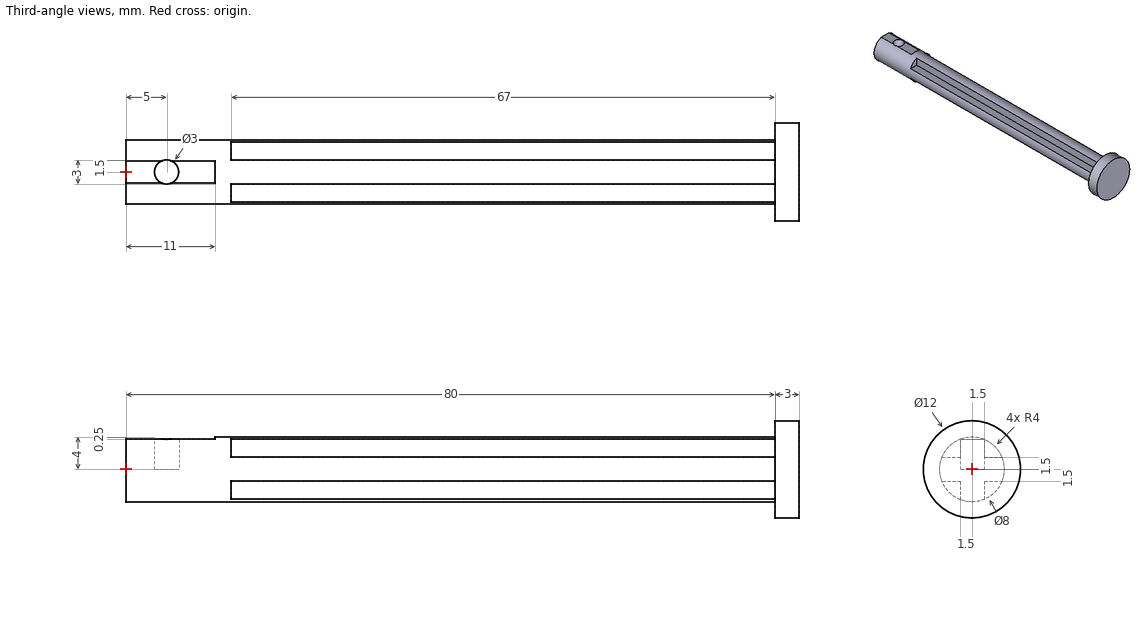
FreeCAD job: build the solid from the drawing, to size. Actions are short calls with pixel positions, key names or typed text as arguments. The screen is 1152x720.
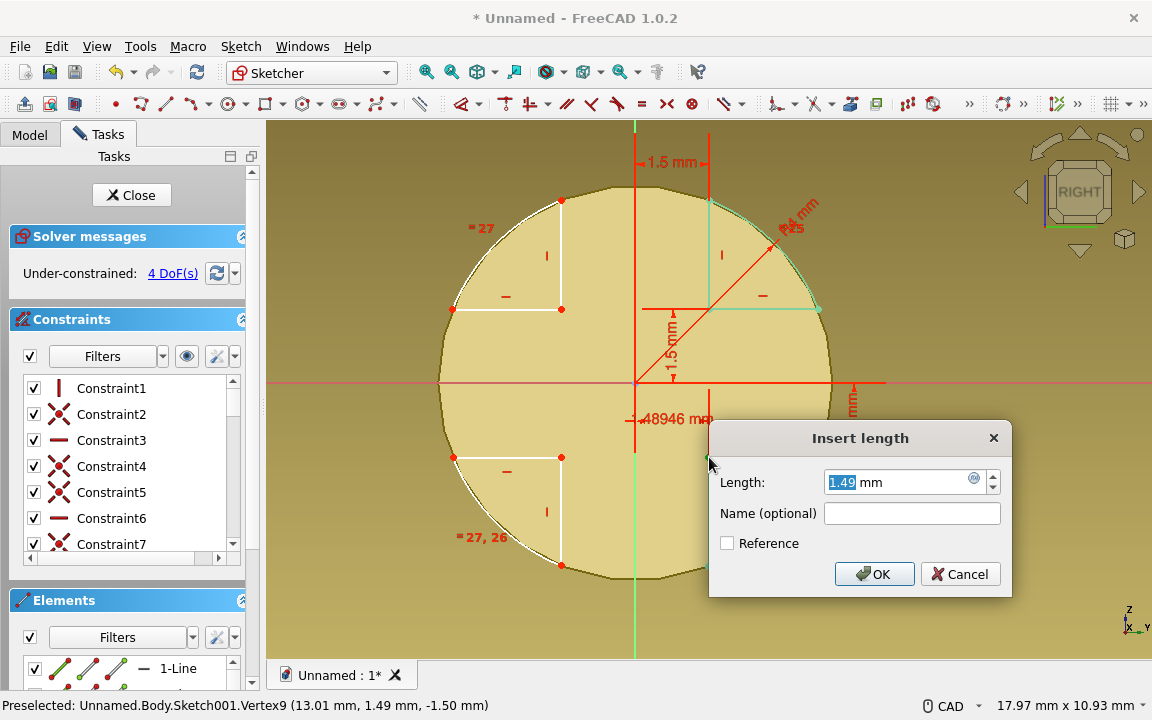
text(1.5)
key(Return)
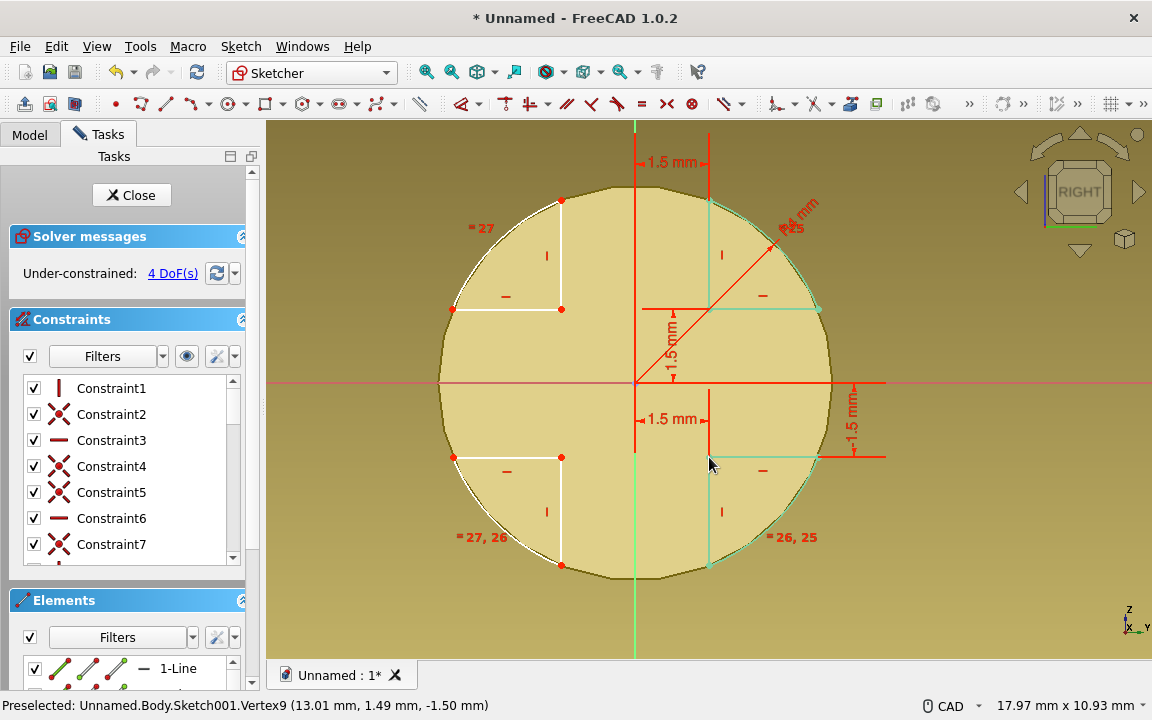
click(561, 566)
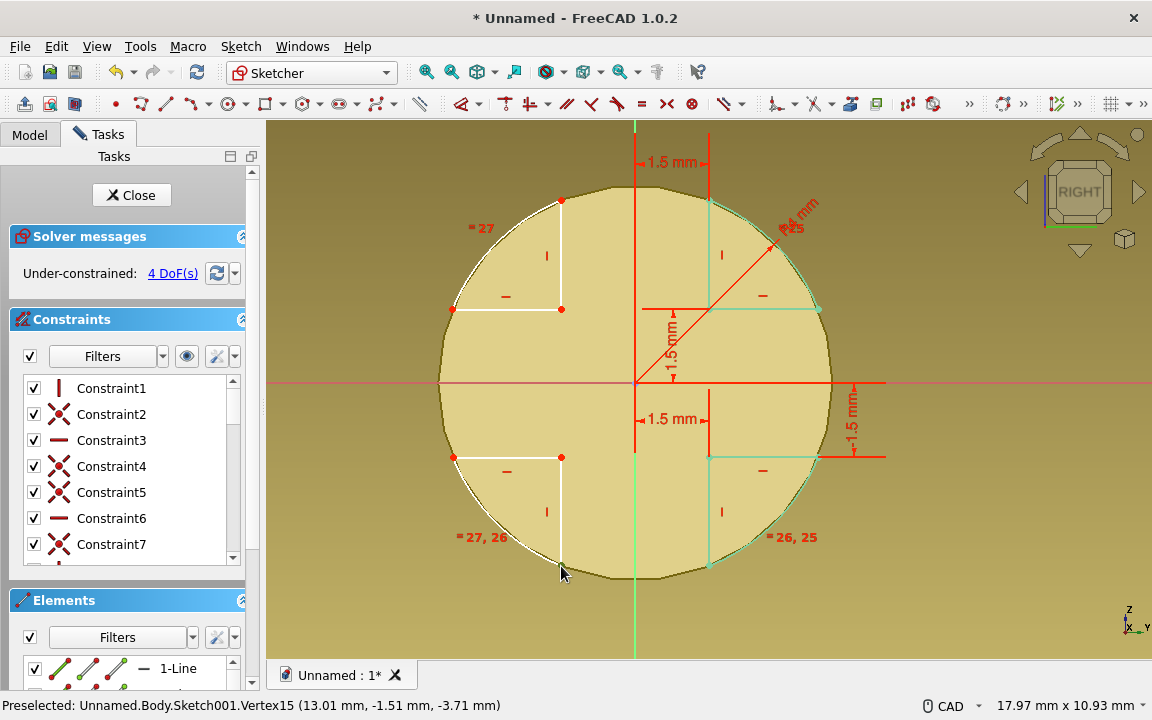
key(l)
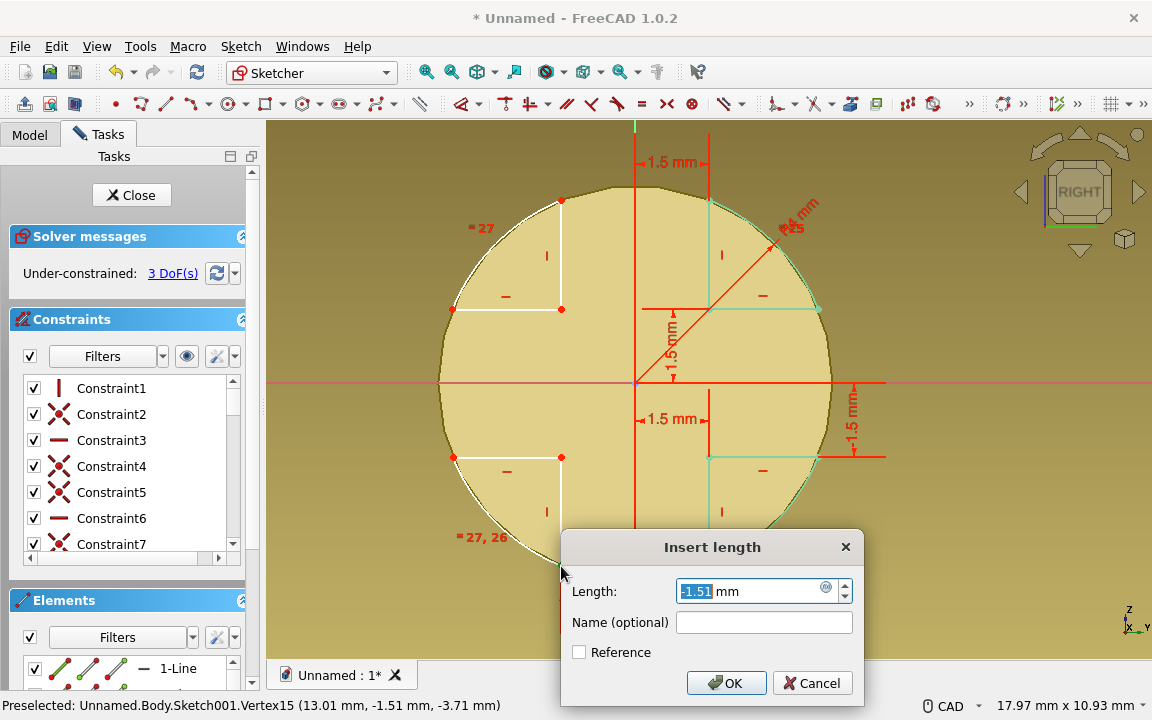
text(-1.5)
key(Return)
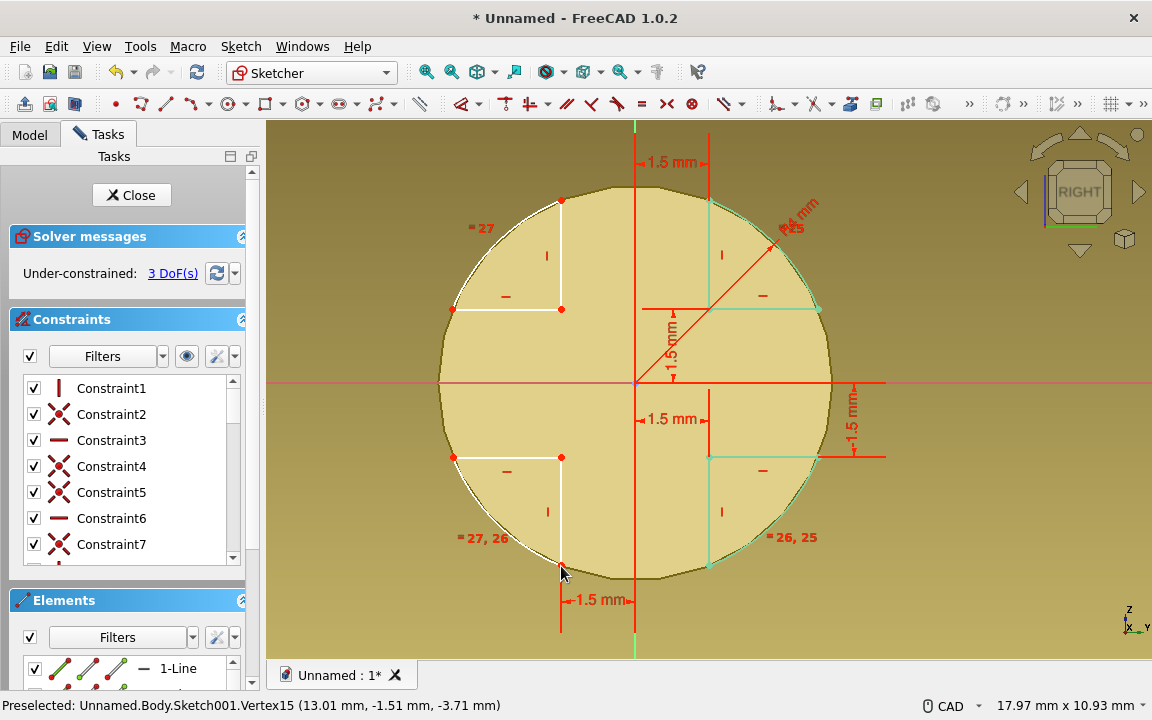
click(561, 458)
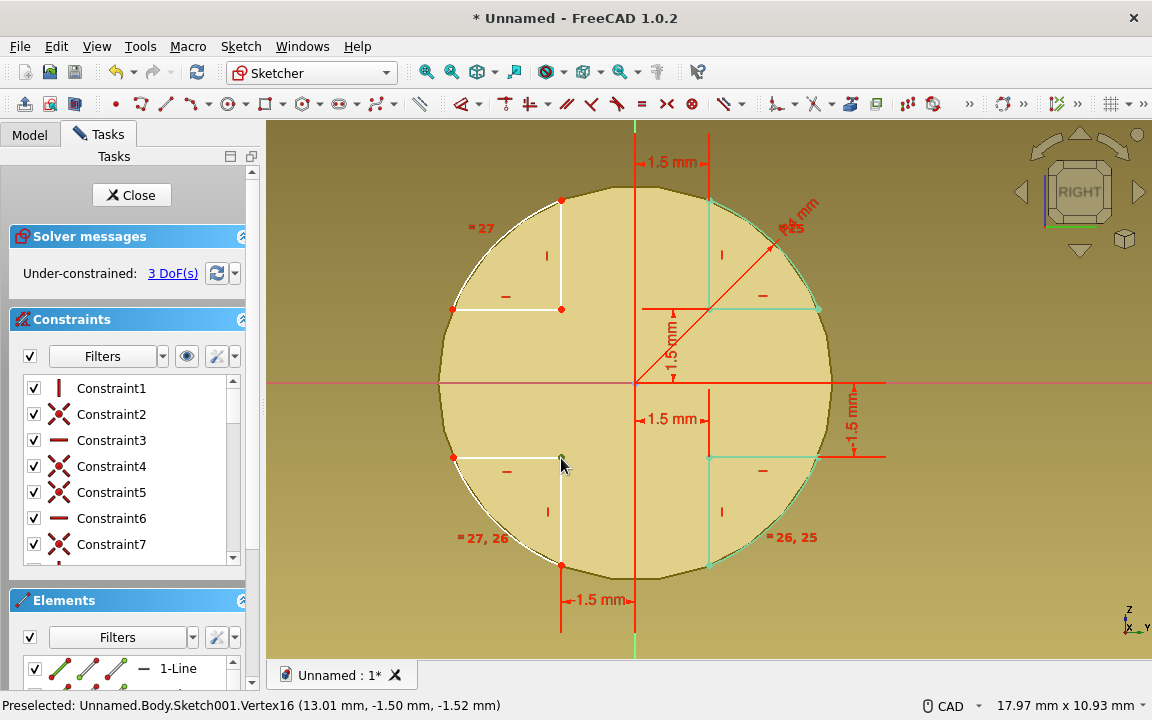
key(i)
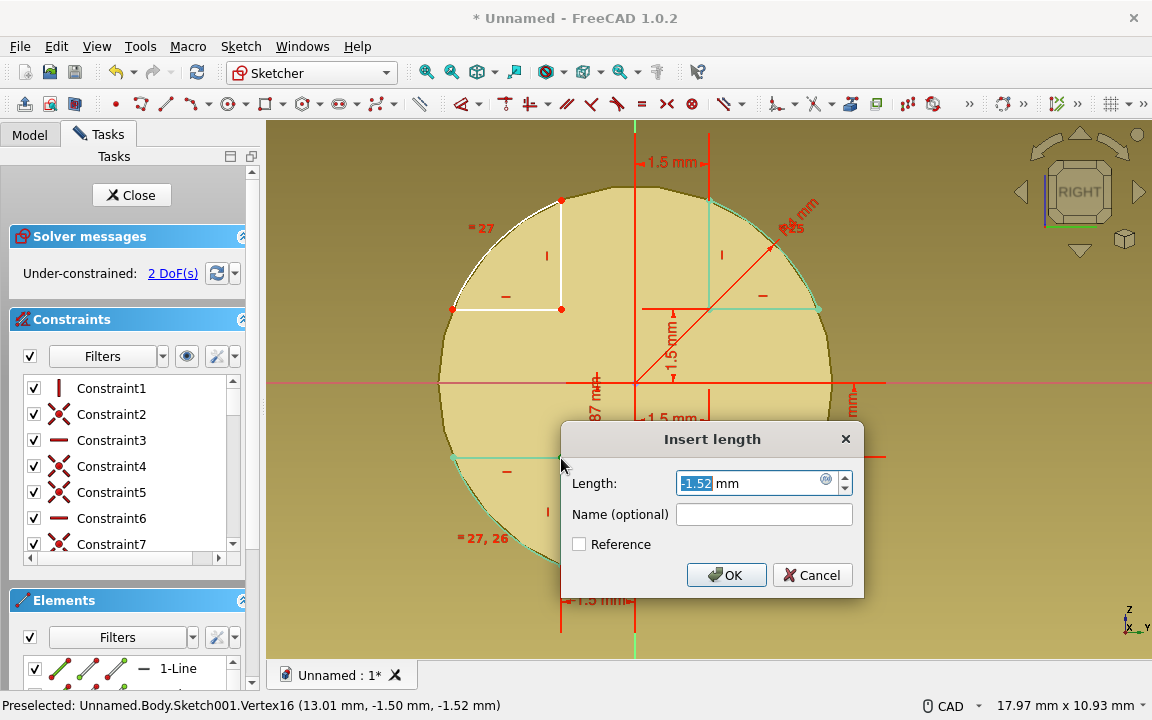
text(-1.5)
key(Return)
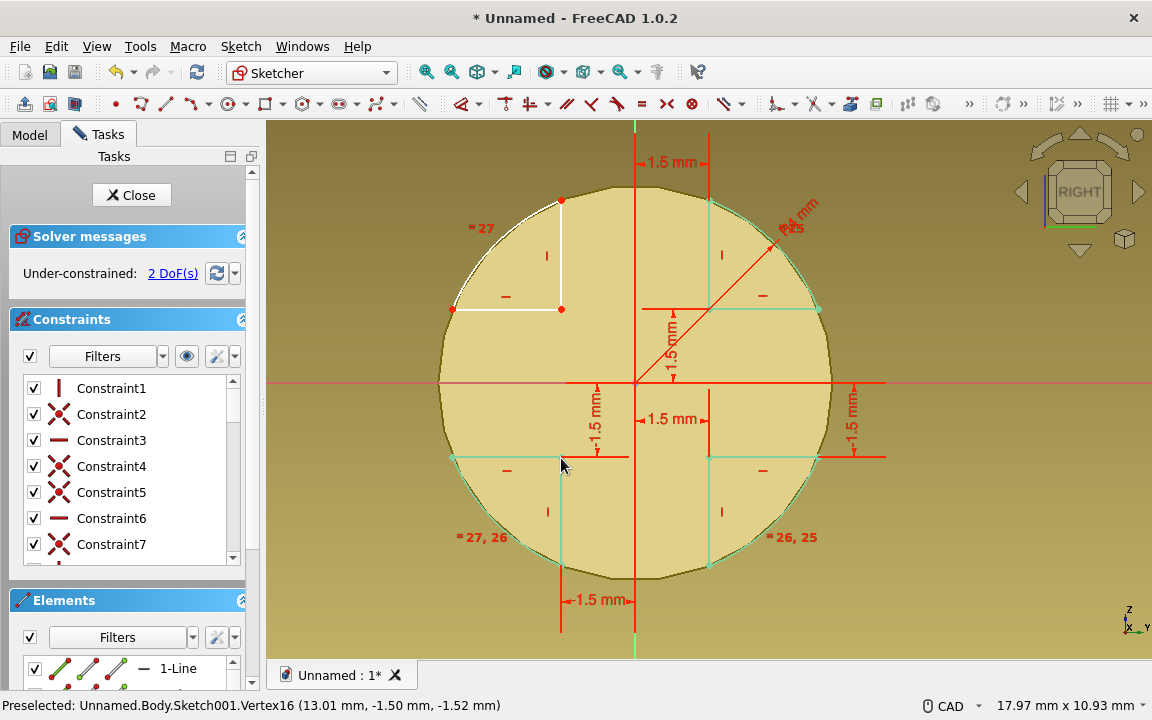
click(452, 310)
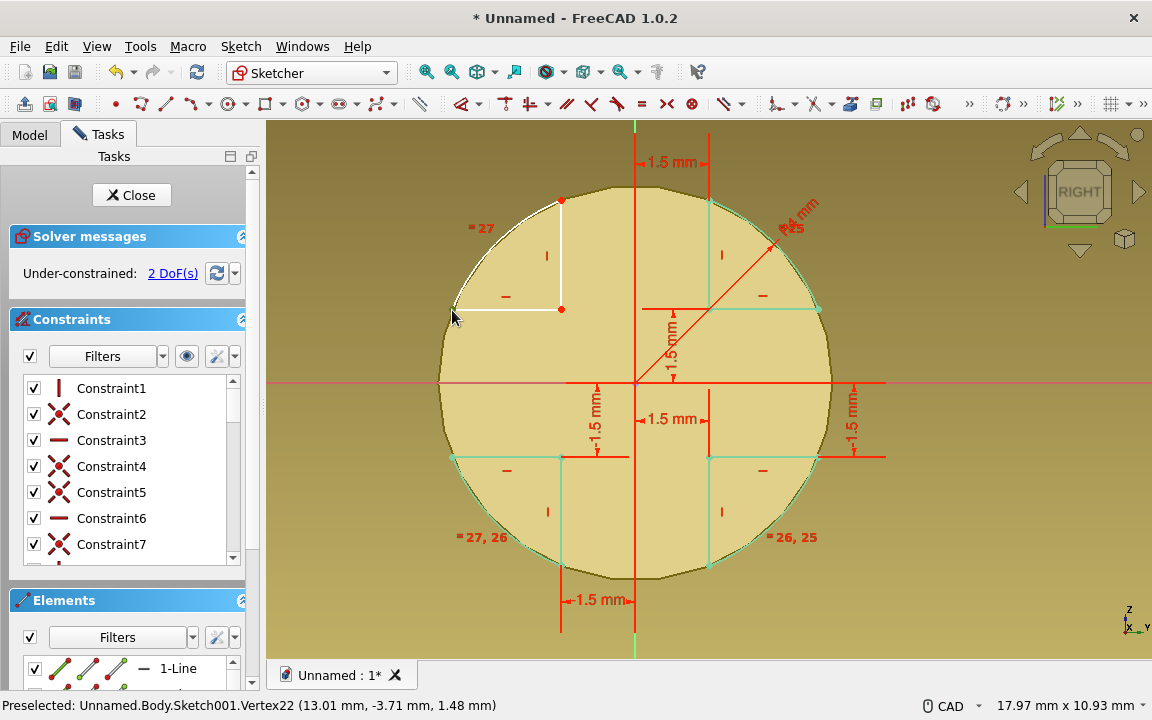
key(i)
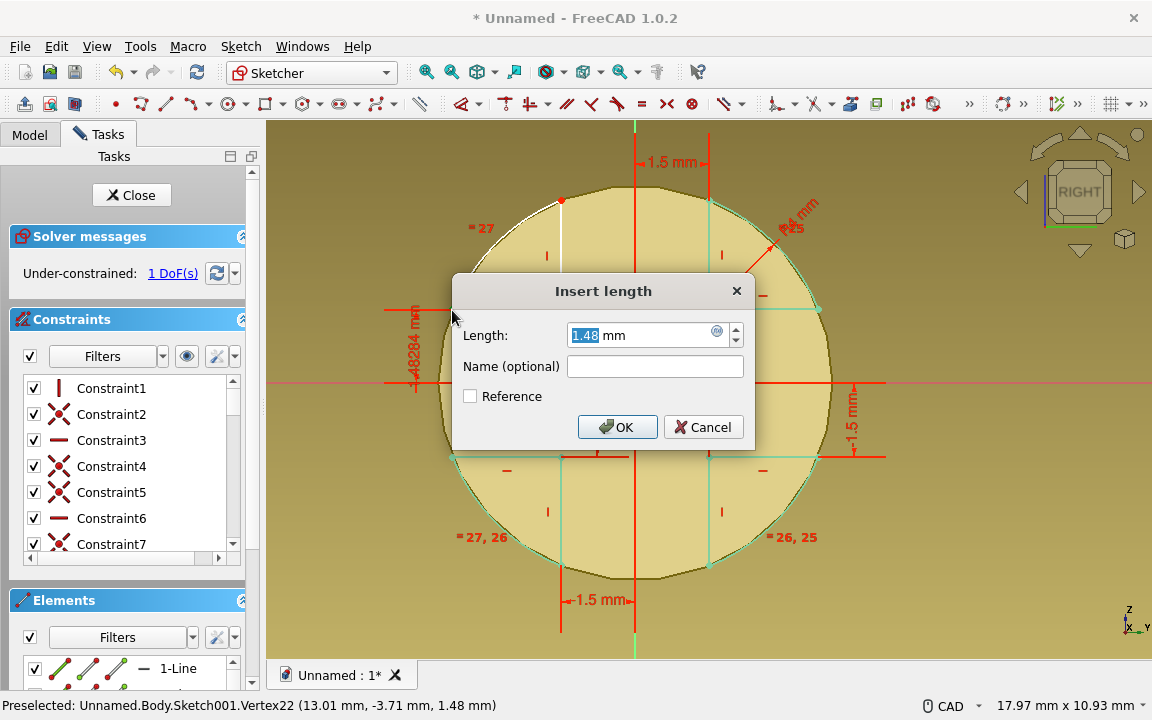
text(1.5)
key(Return)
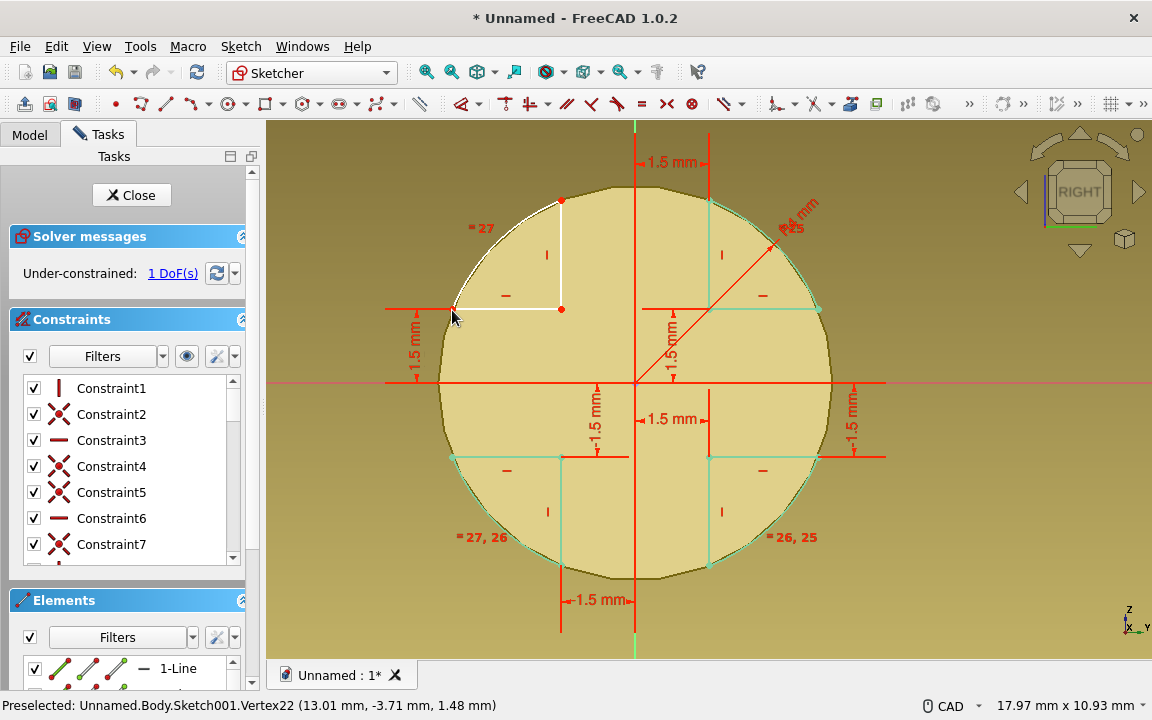
click(561, 309)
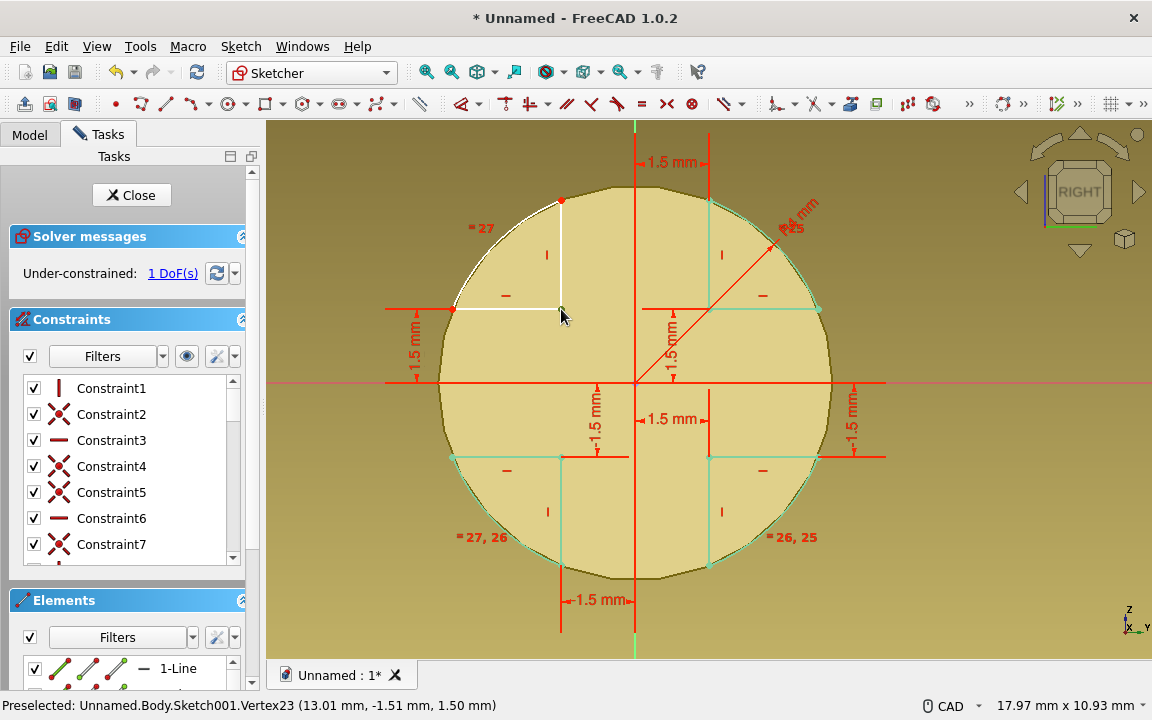
key(l)